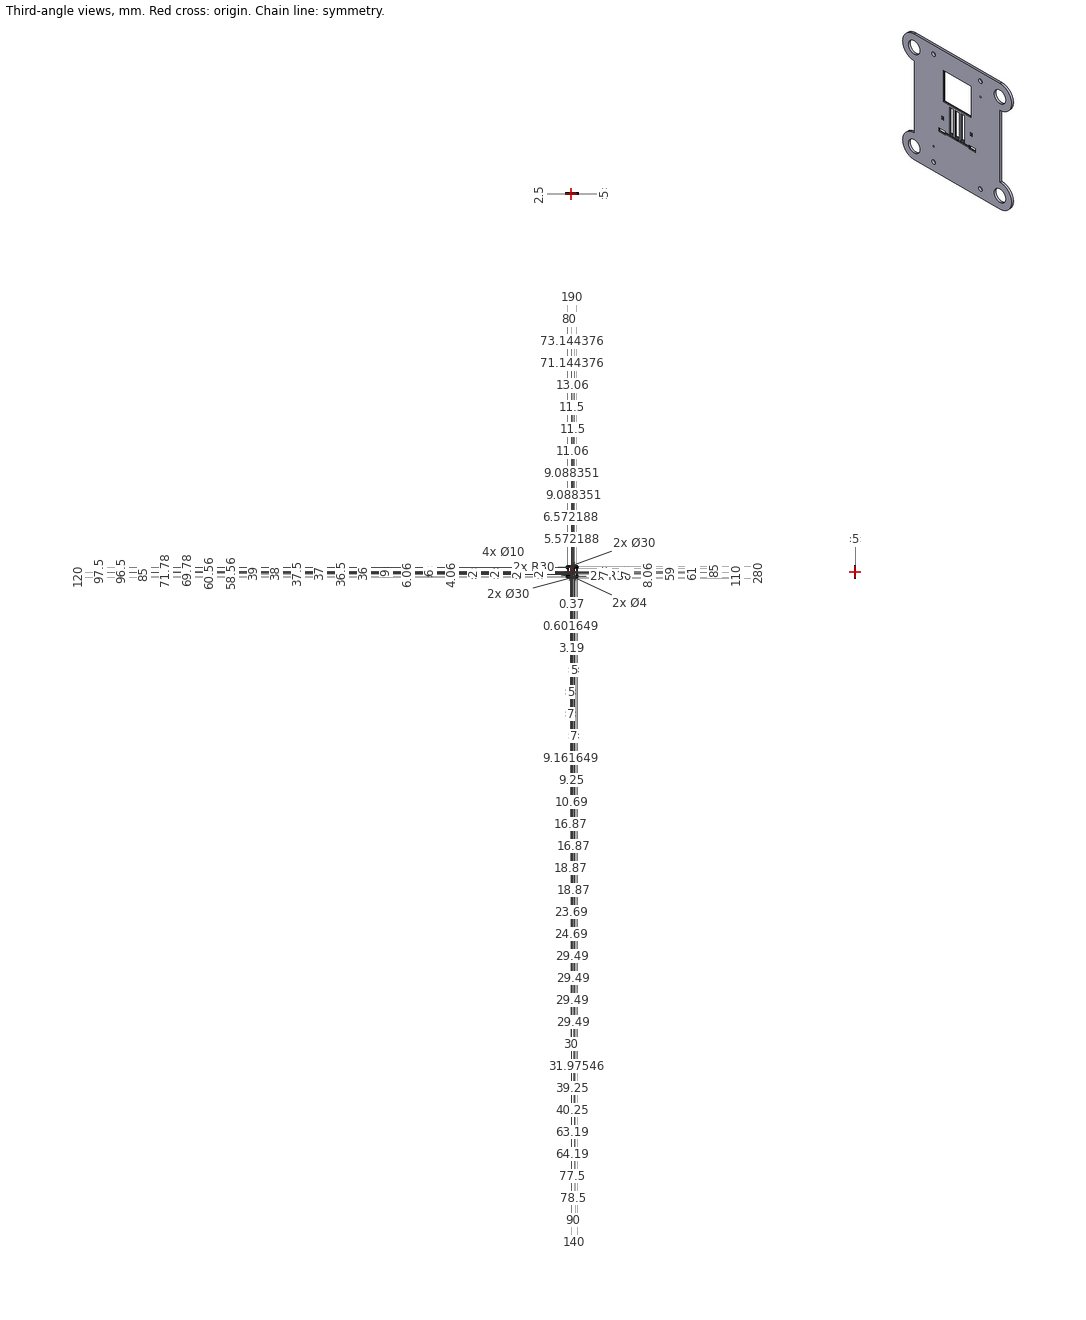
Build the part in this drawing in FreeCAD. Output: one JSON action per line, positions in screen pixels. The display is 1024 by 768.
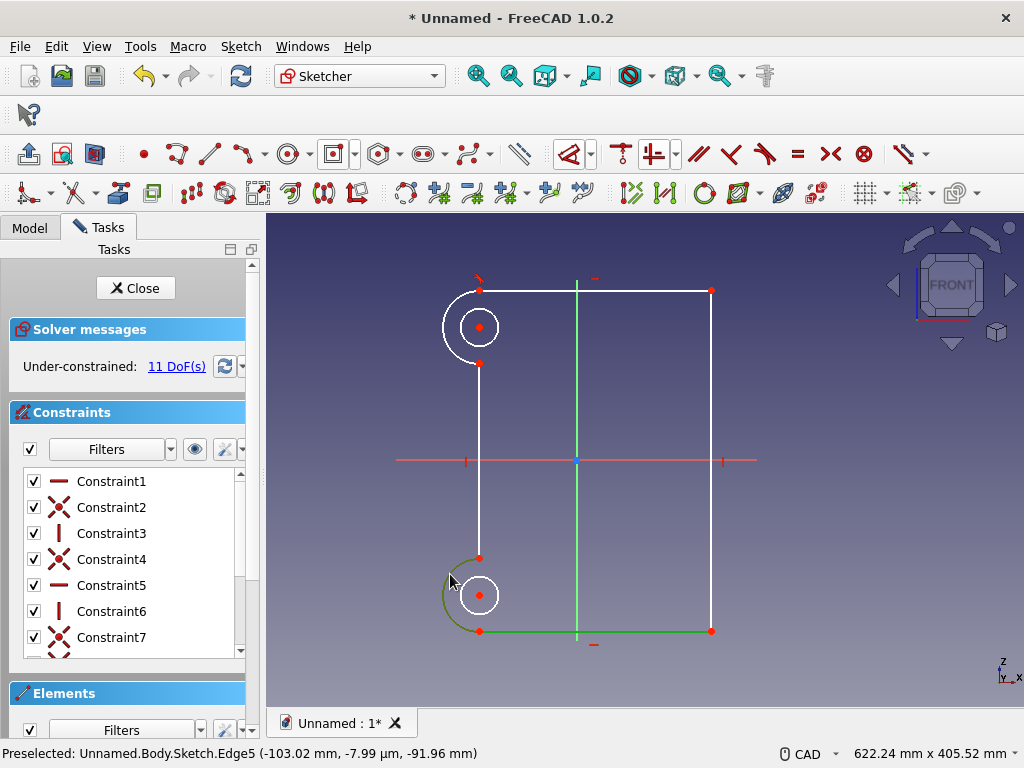
{"action": "left_click", "coordinate": [765, 154]}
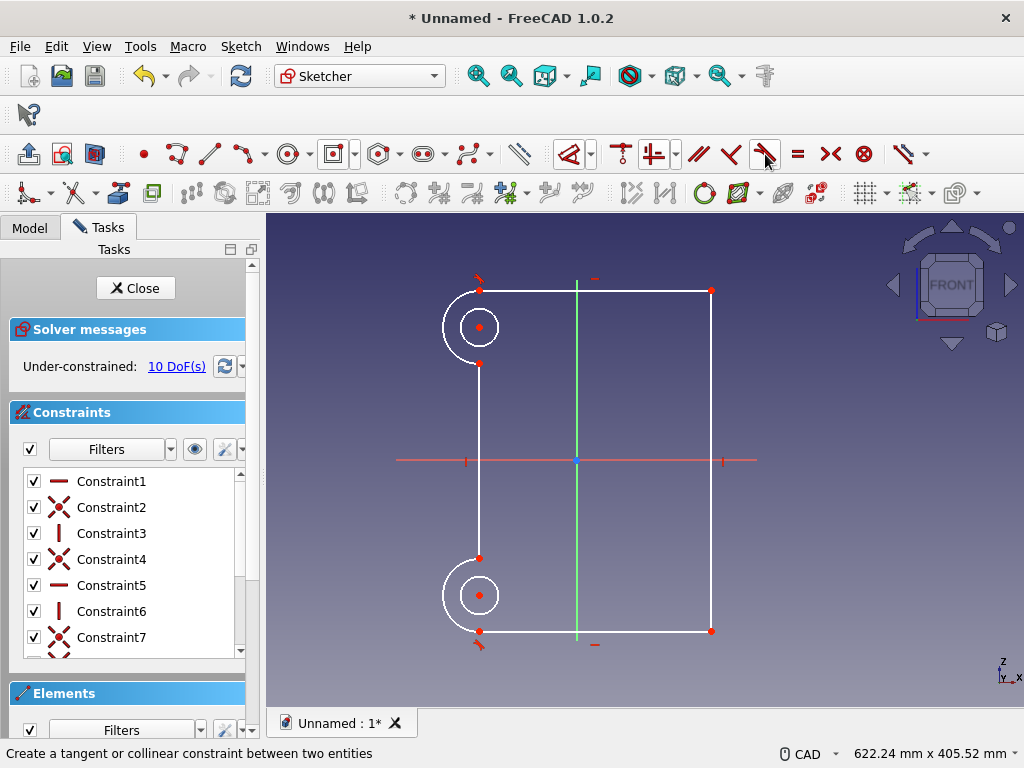
{"action": "left_click", "coordinate": [450, 574]}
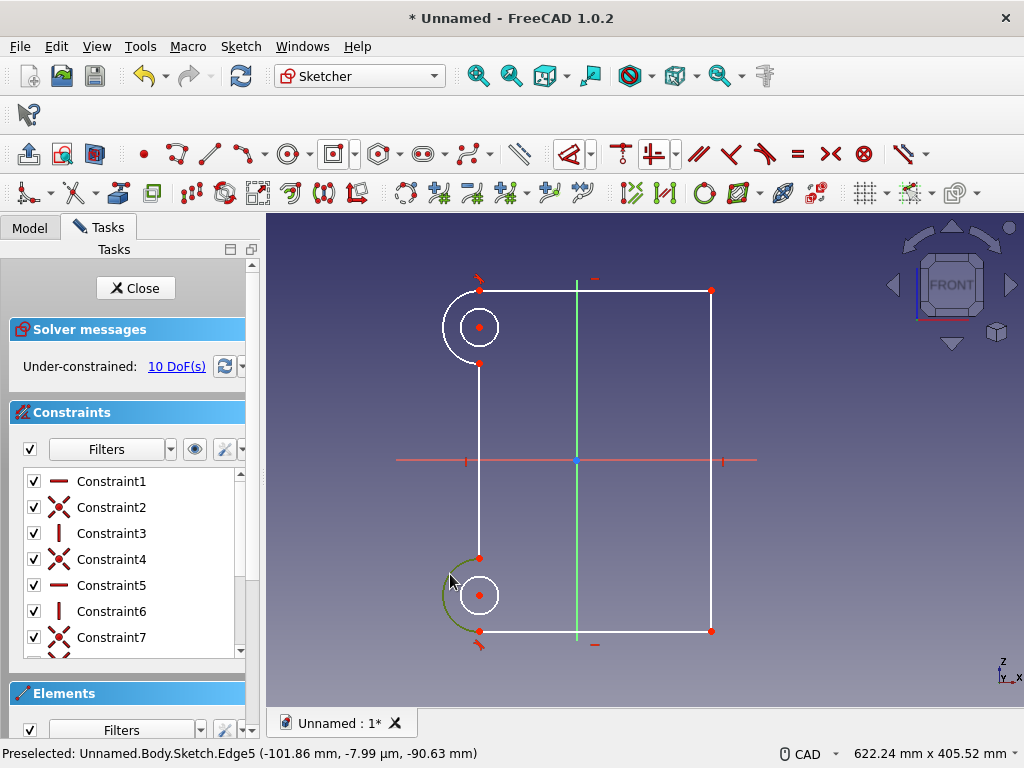
{"action": "left_click", "coordinate": [450, 306]}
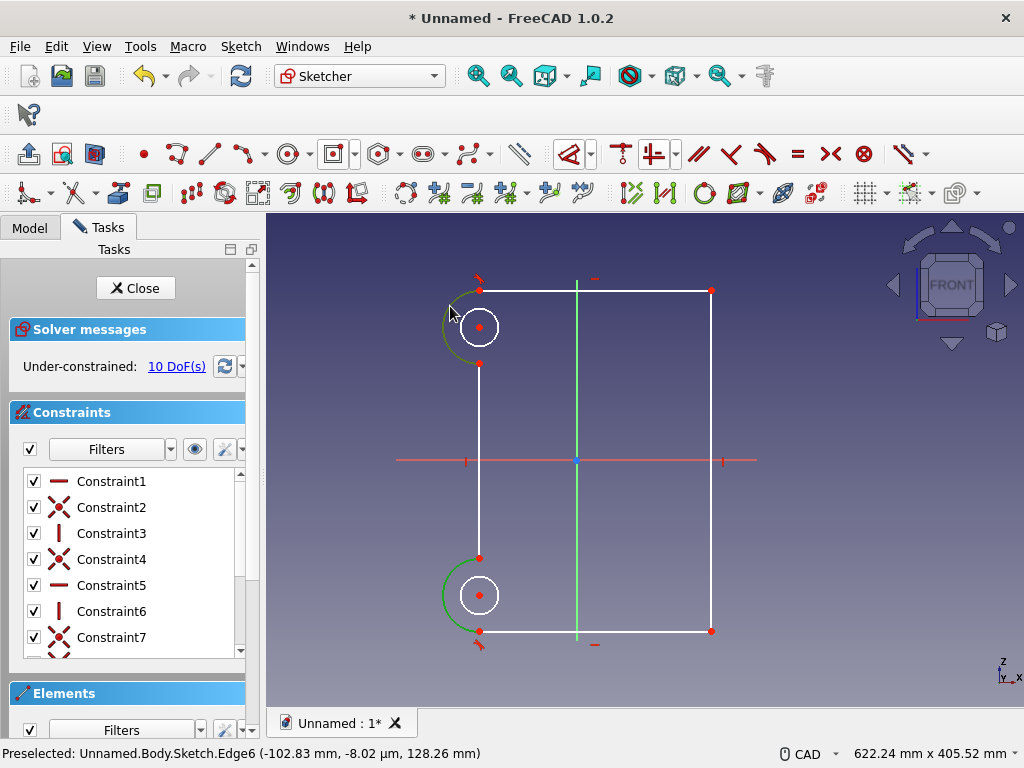
{"action": "left_click", "coordinate": [798, 154]}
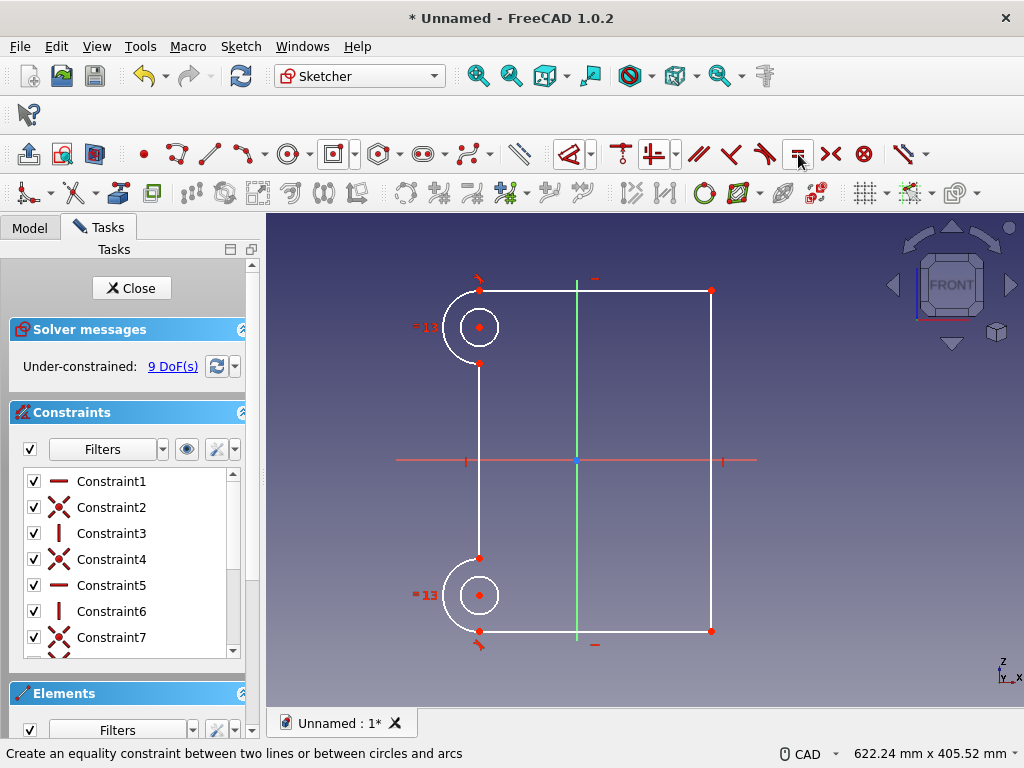
{"action": "left_click", "coordinate": [493, 314]}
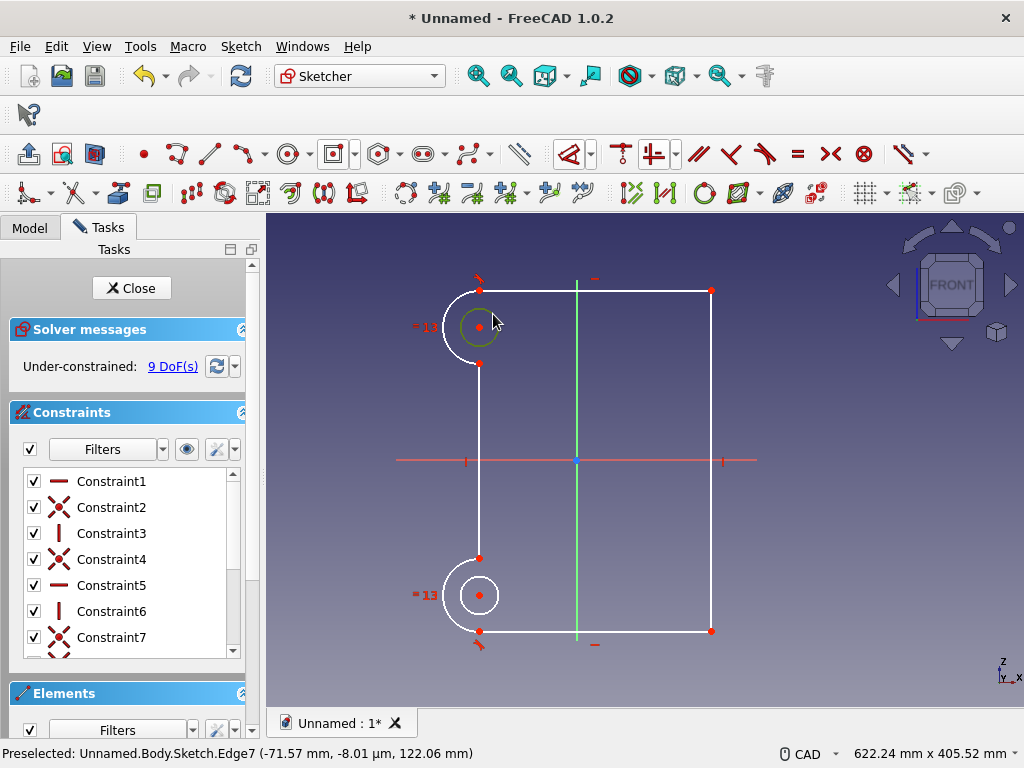
{"action": "left_click", "coordinate": [493, 582]}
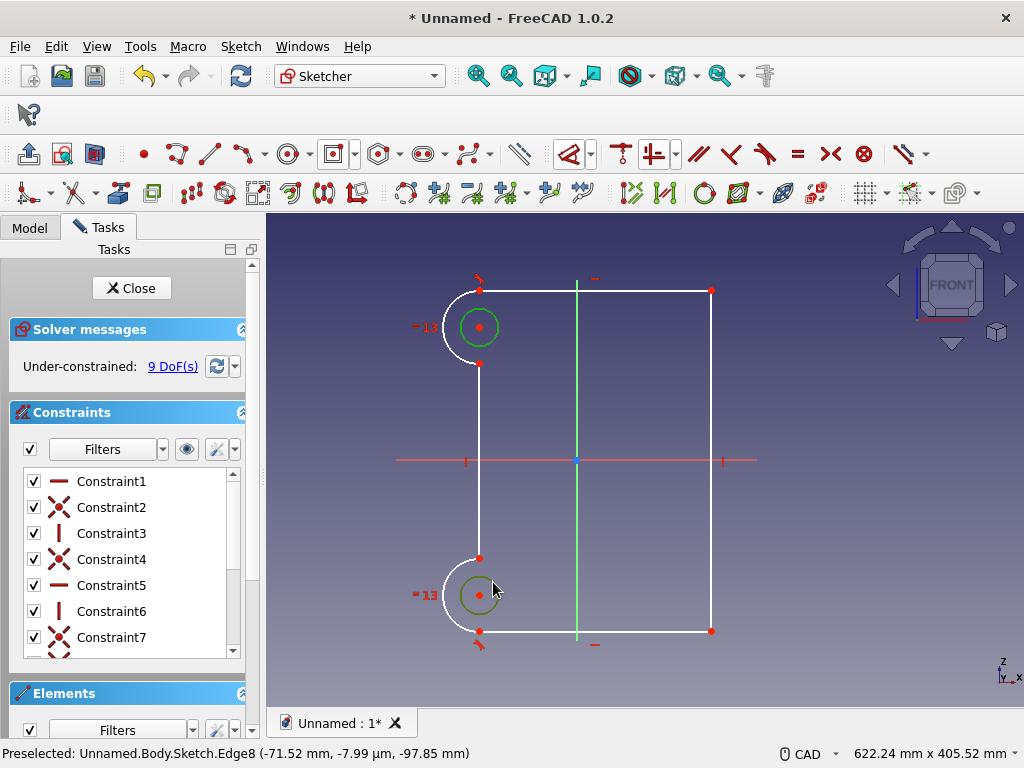
{"action": "left_click", "coordinate": [798, 154]}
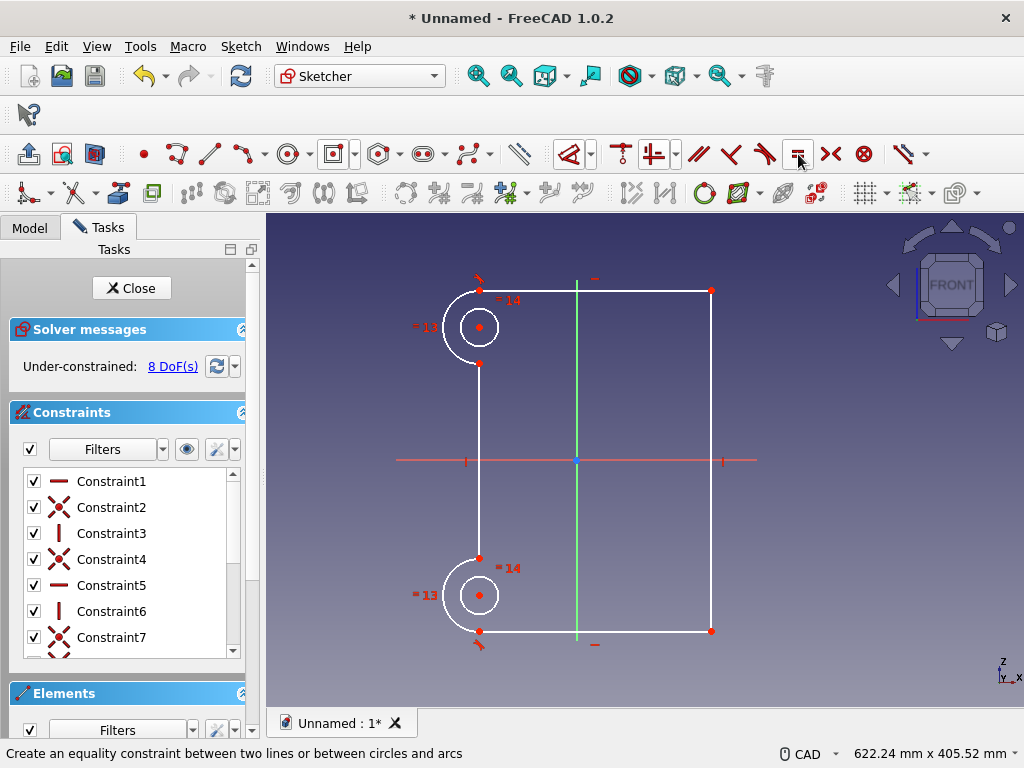
{"action": "left_click", "coordinate": [479, 595]}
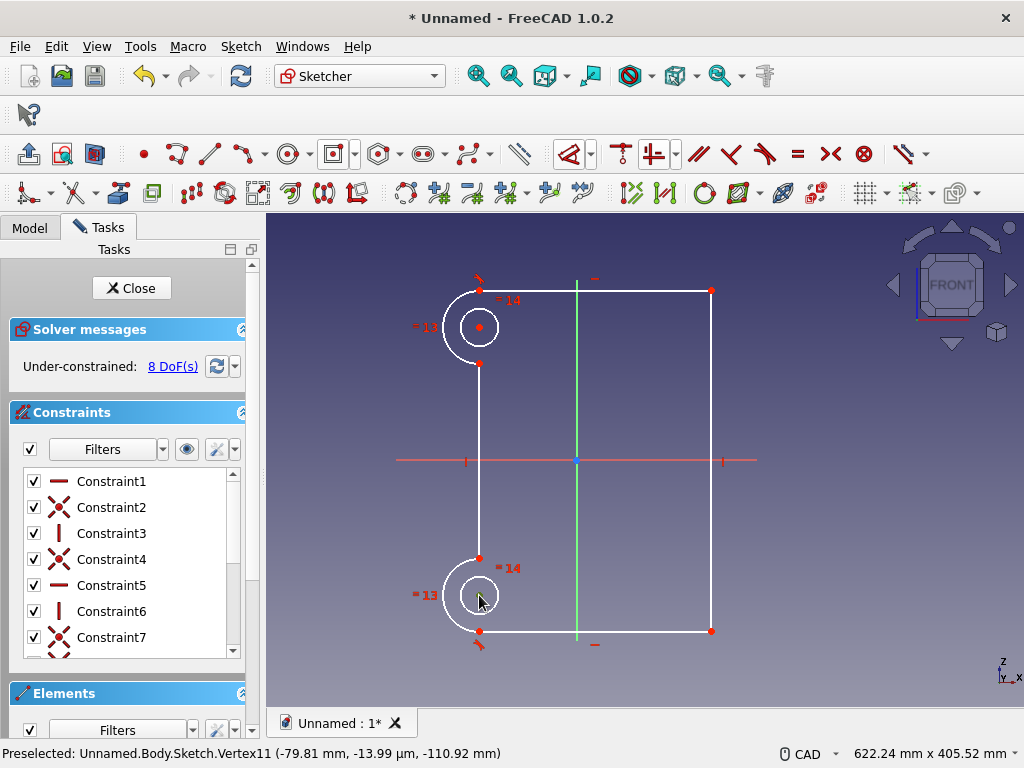
{"action": "left_click", "coordinate": [479, 328]}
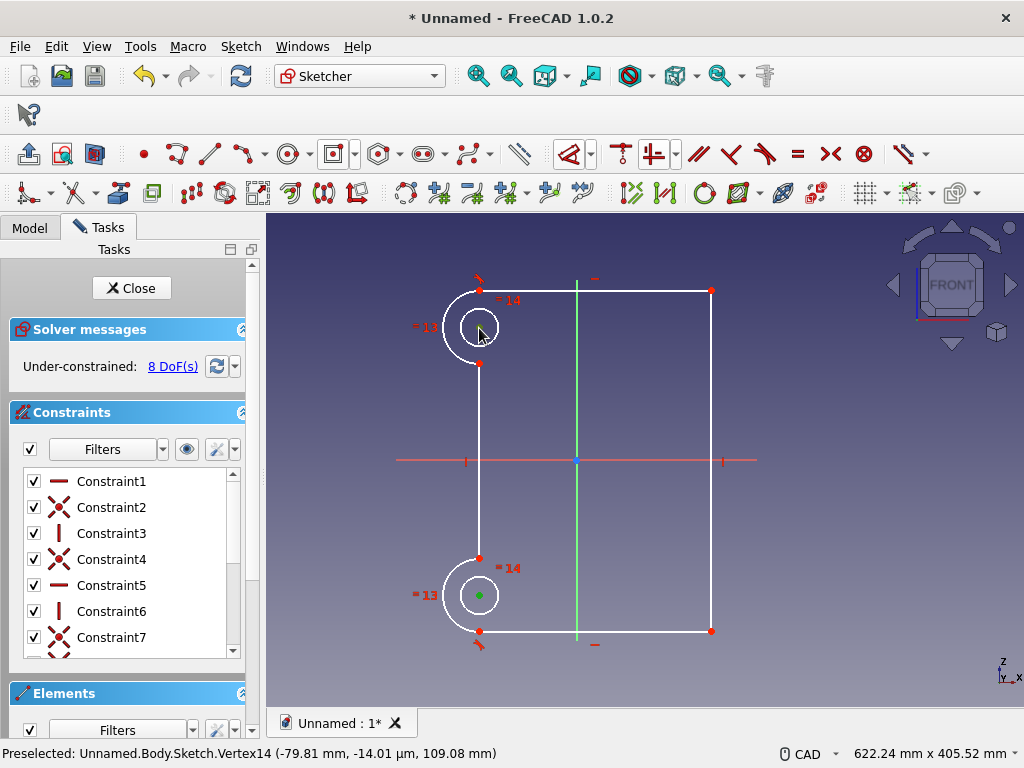
{"action": "left_click", "coordinate": [415, 460]}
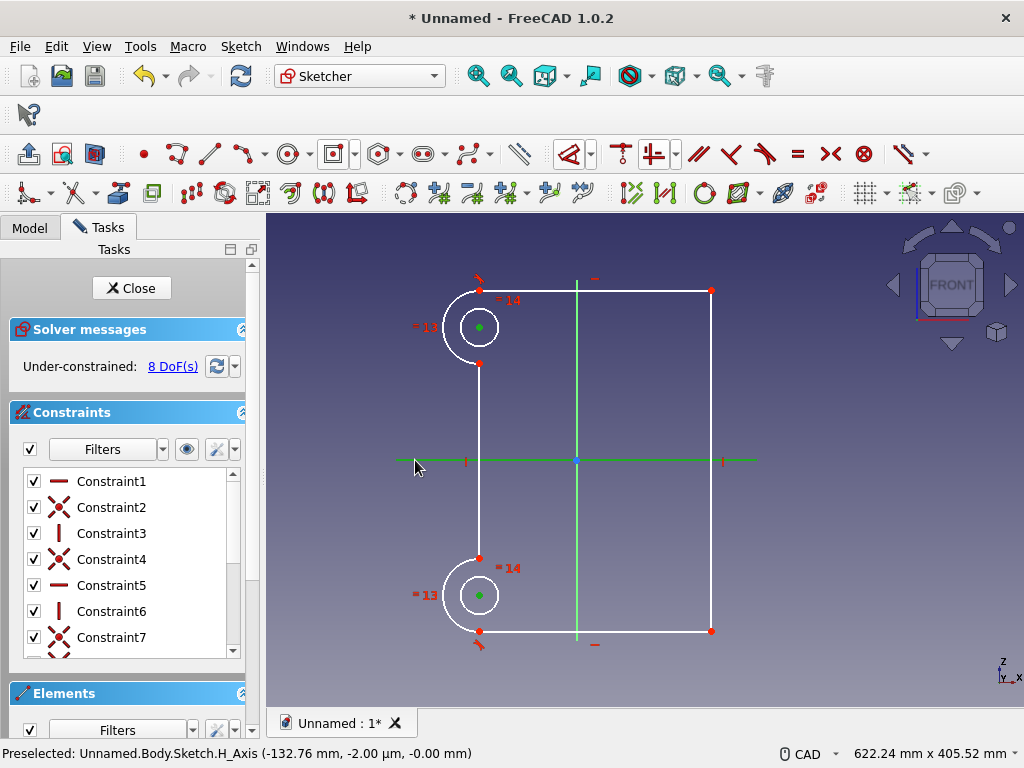
{"action": "left_click", "coordinate": [831, 154]}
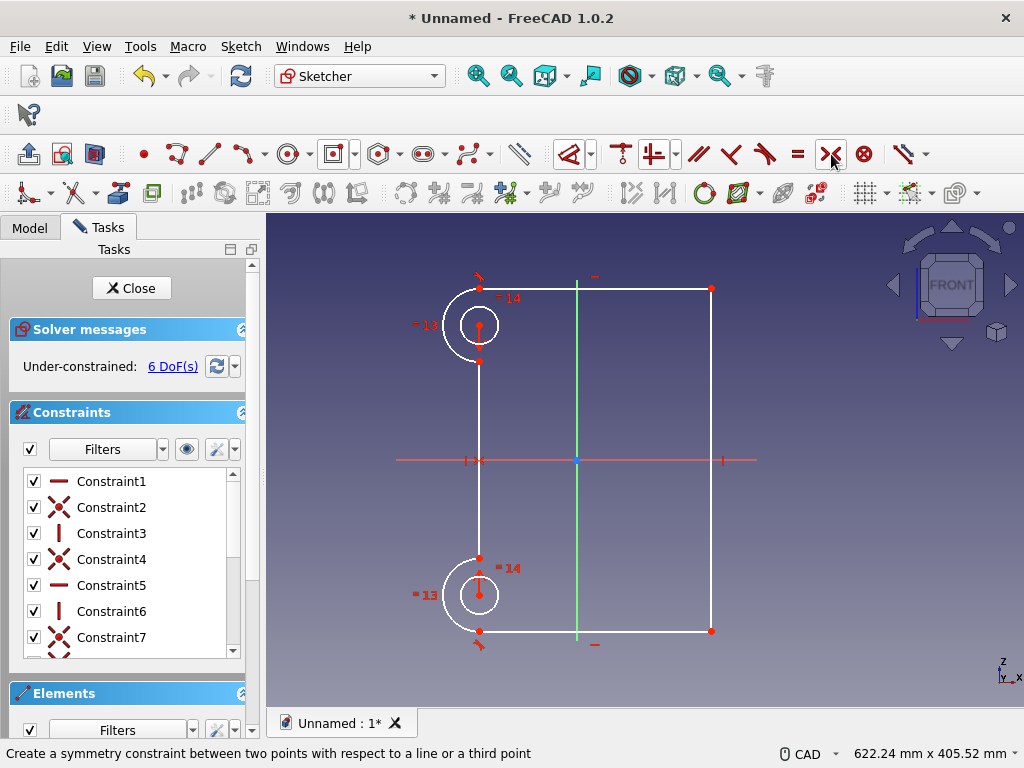
{"action": "left_click", "coordinate": [450, 574]}